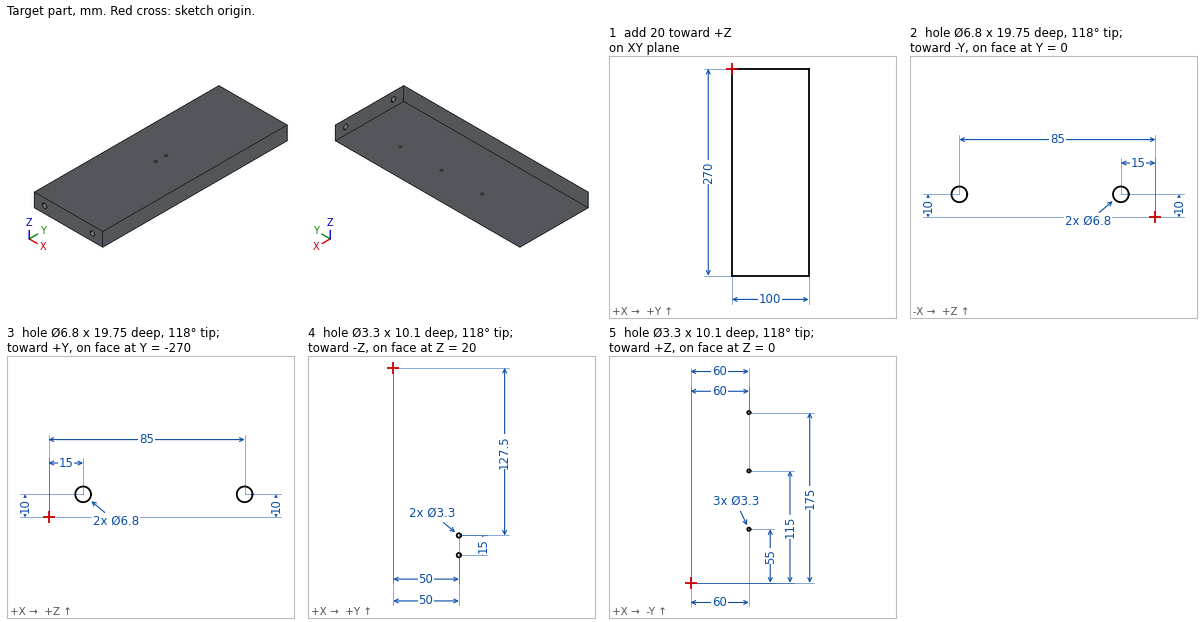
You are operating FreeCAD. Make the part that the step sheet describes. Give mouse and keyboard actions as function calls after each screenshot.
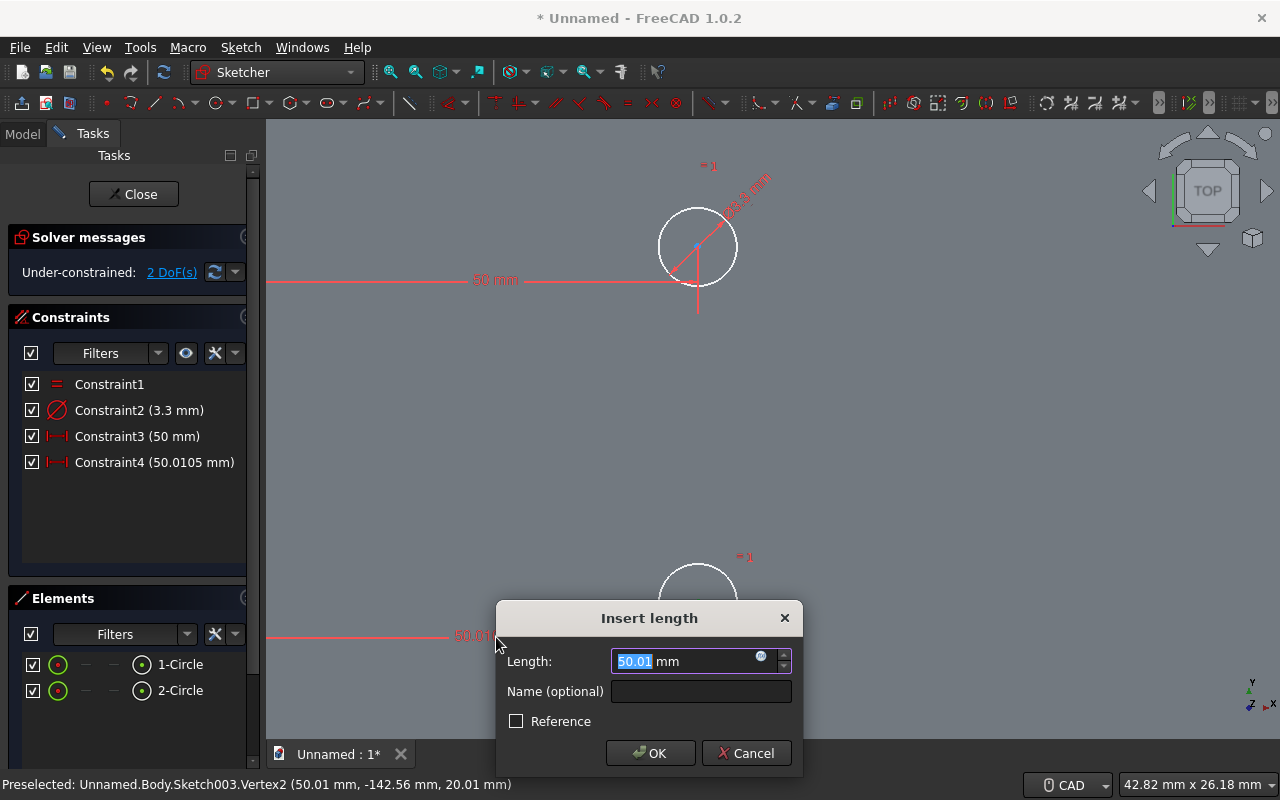
text(50)
key(Return)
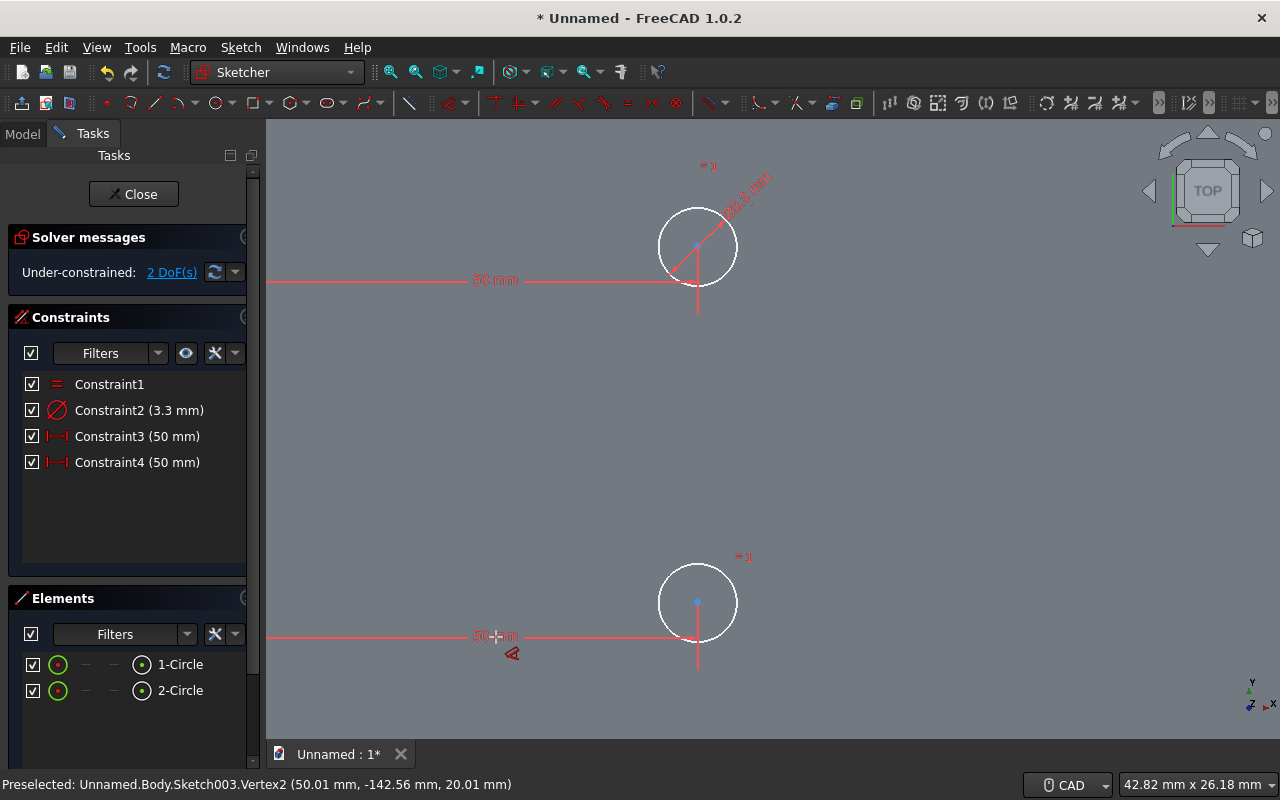
click(698, 247)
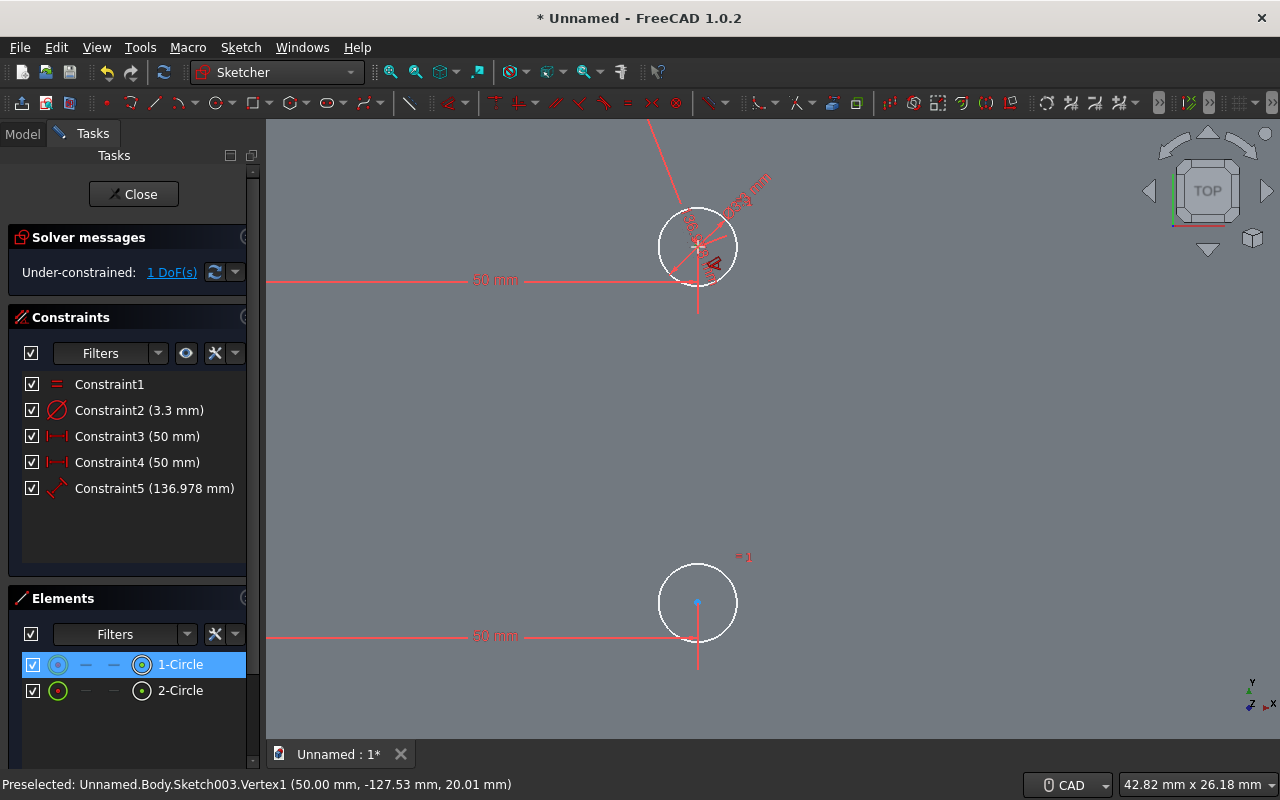
click(698, 603)
click(732, 425)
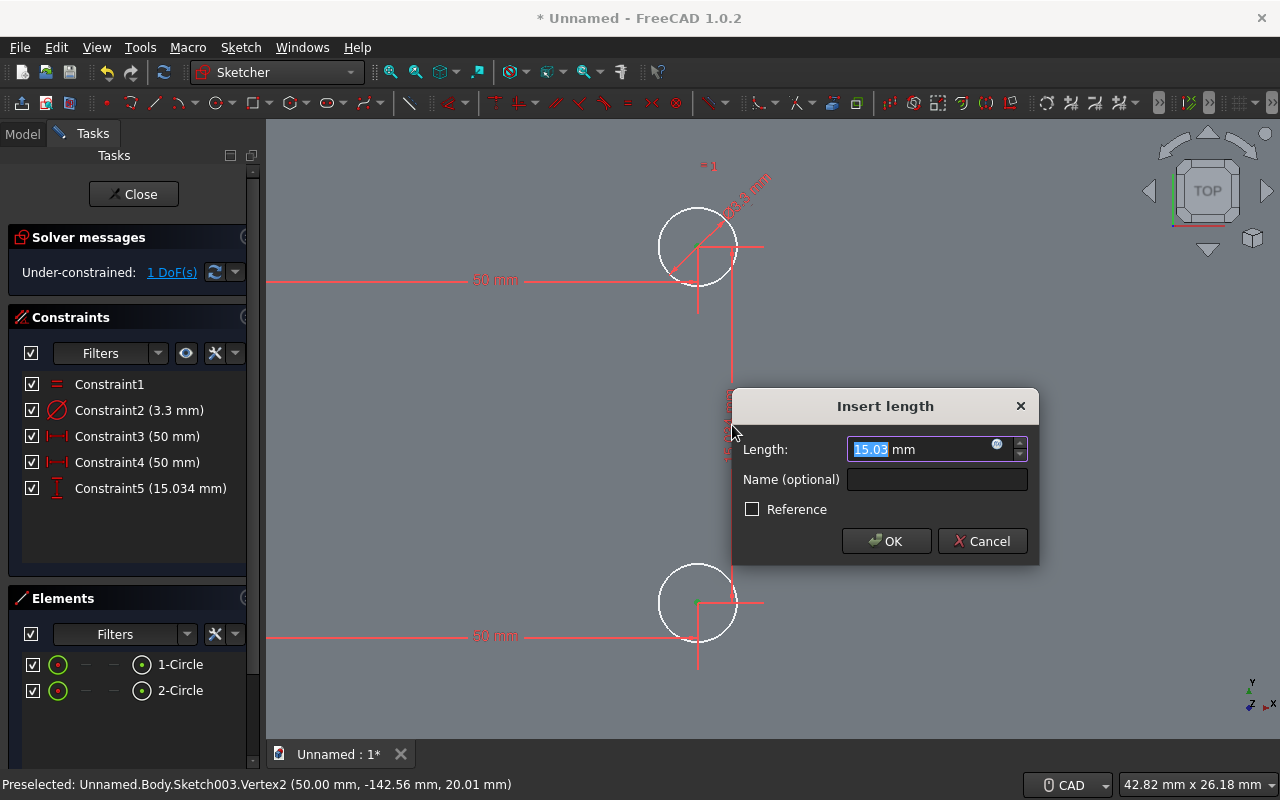
text(15)
key(Return)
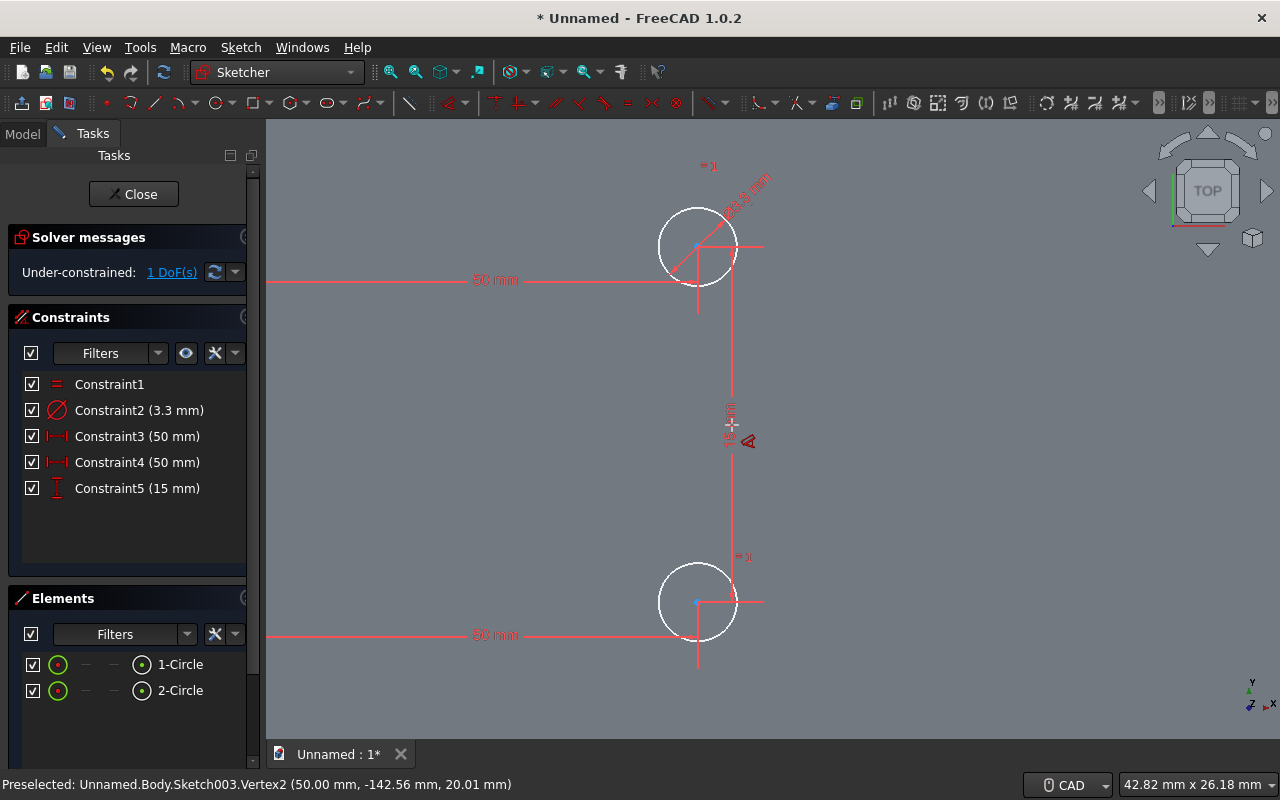
click(698, 247)
click(732, 174)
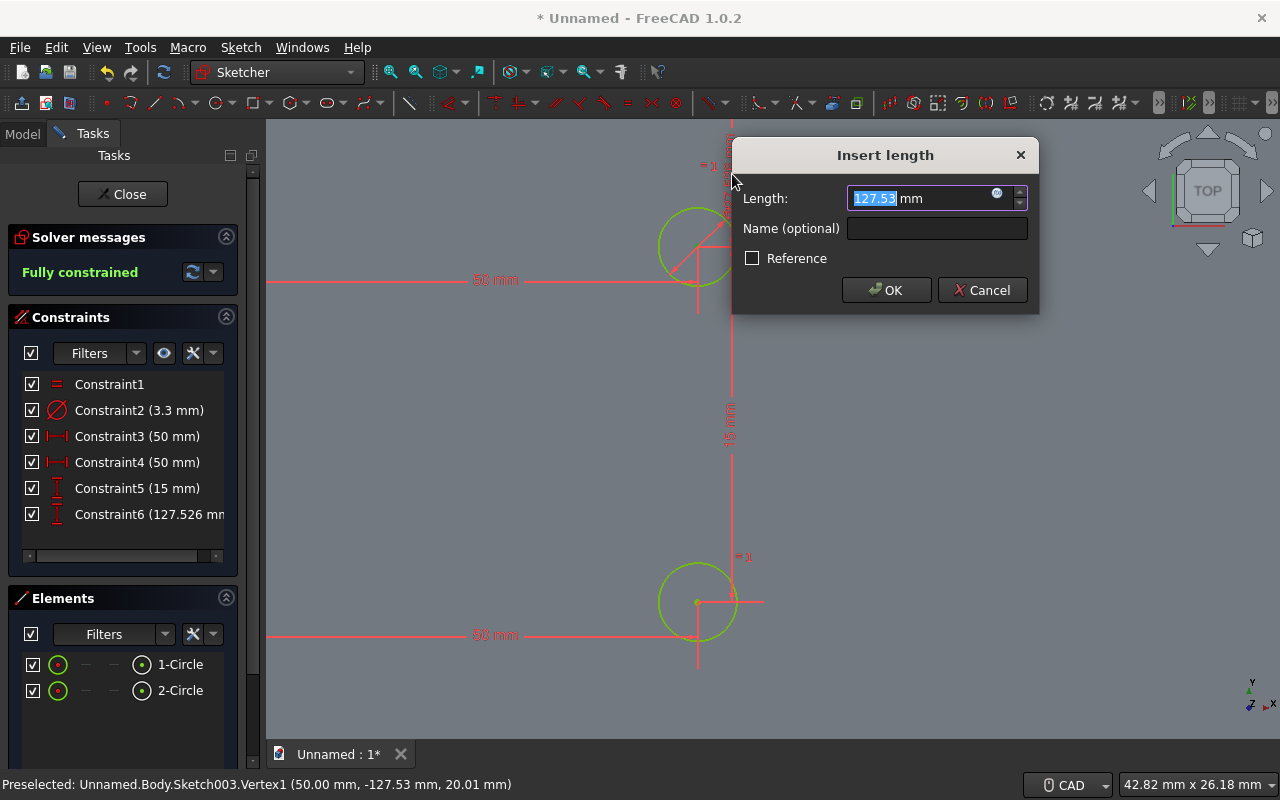
text(127.5)
key(Return)
key(Escape)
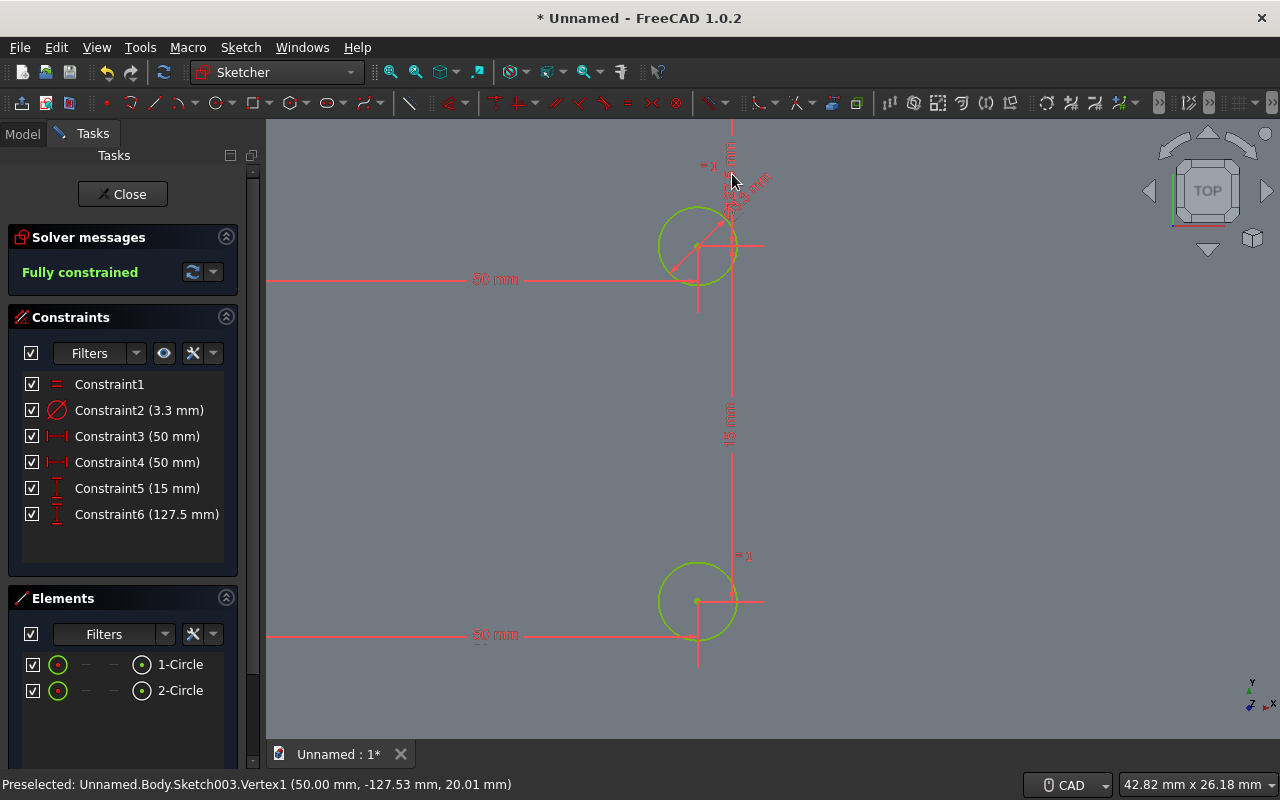
click(123, 194)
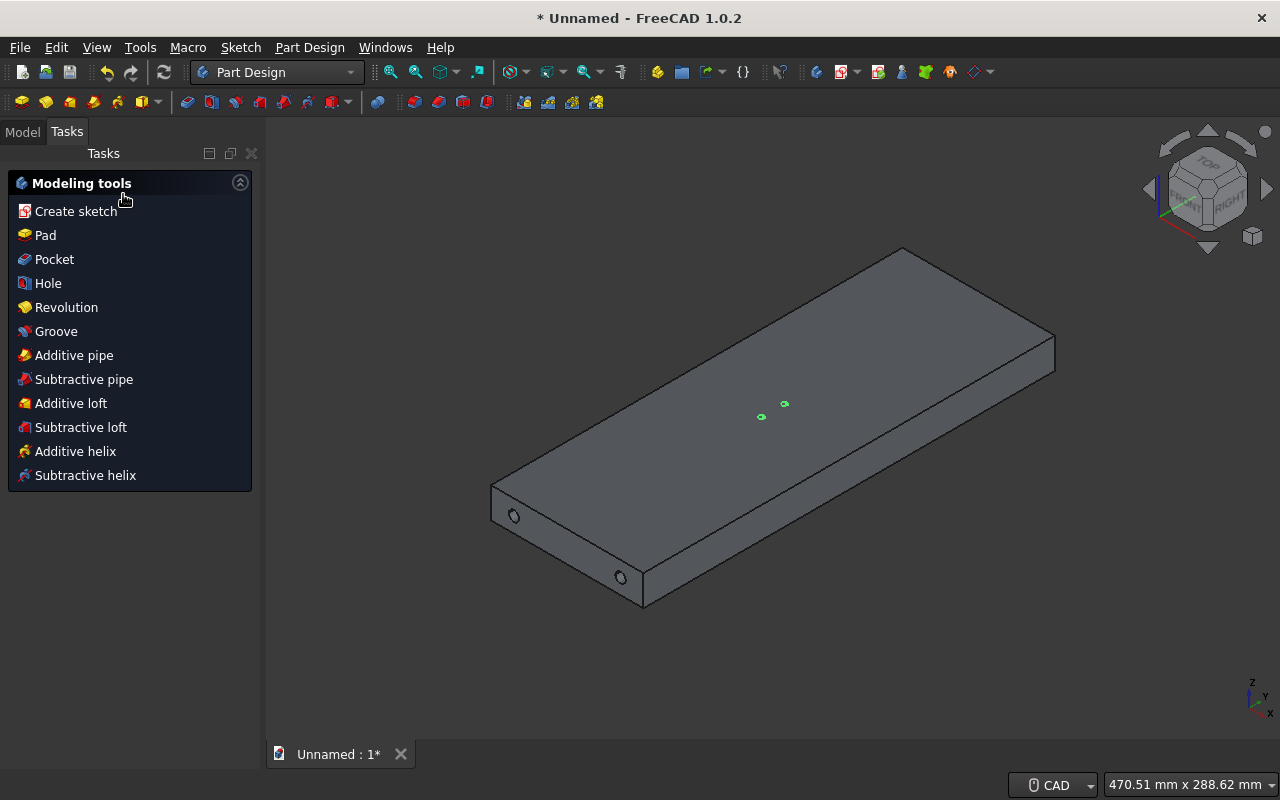
click(212, 102)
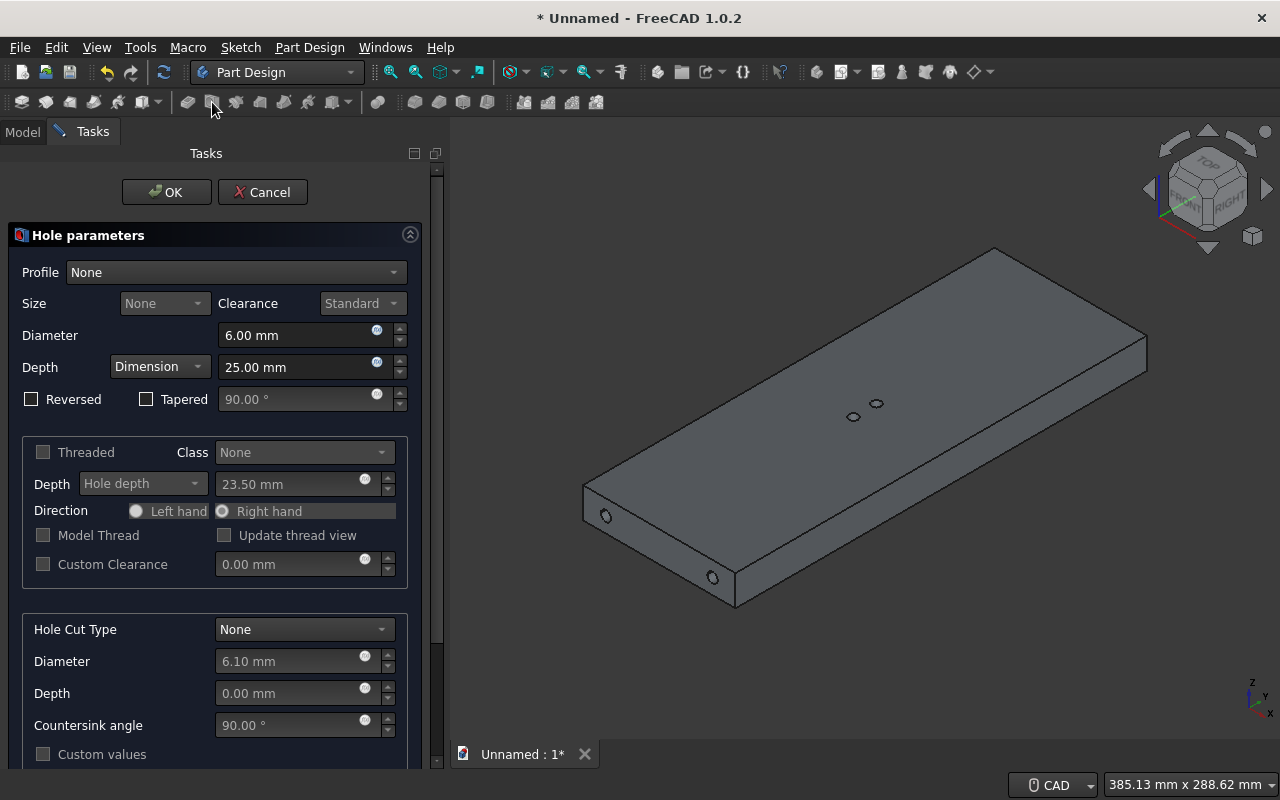
triple_click(305, 335)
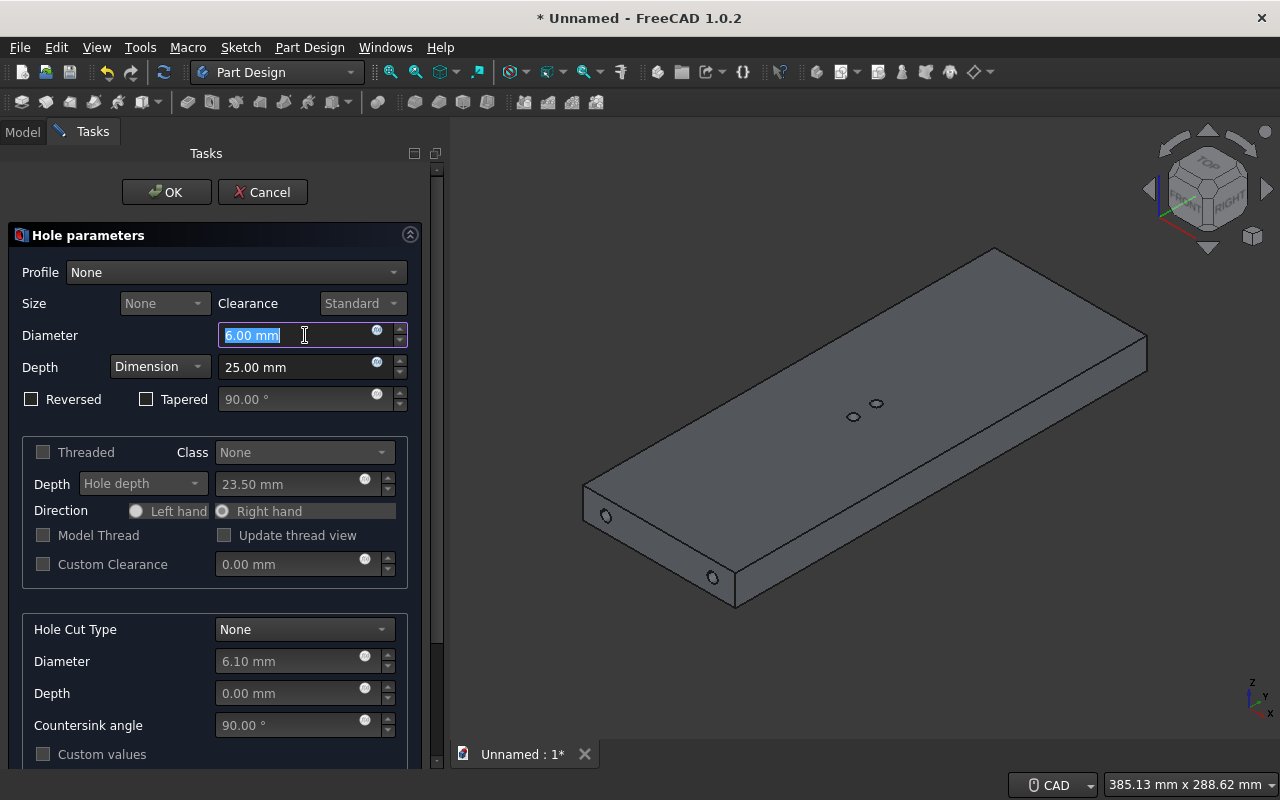
text(3.3)
key(Tab)